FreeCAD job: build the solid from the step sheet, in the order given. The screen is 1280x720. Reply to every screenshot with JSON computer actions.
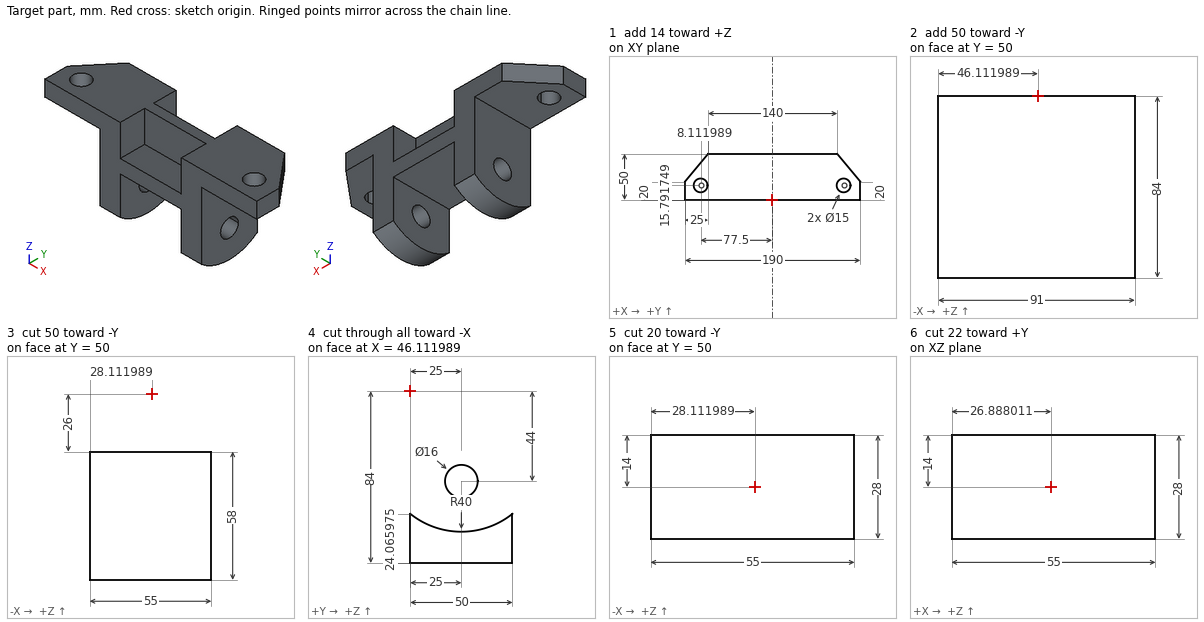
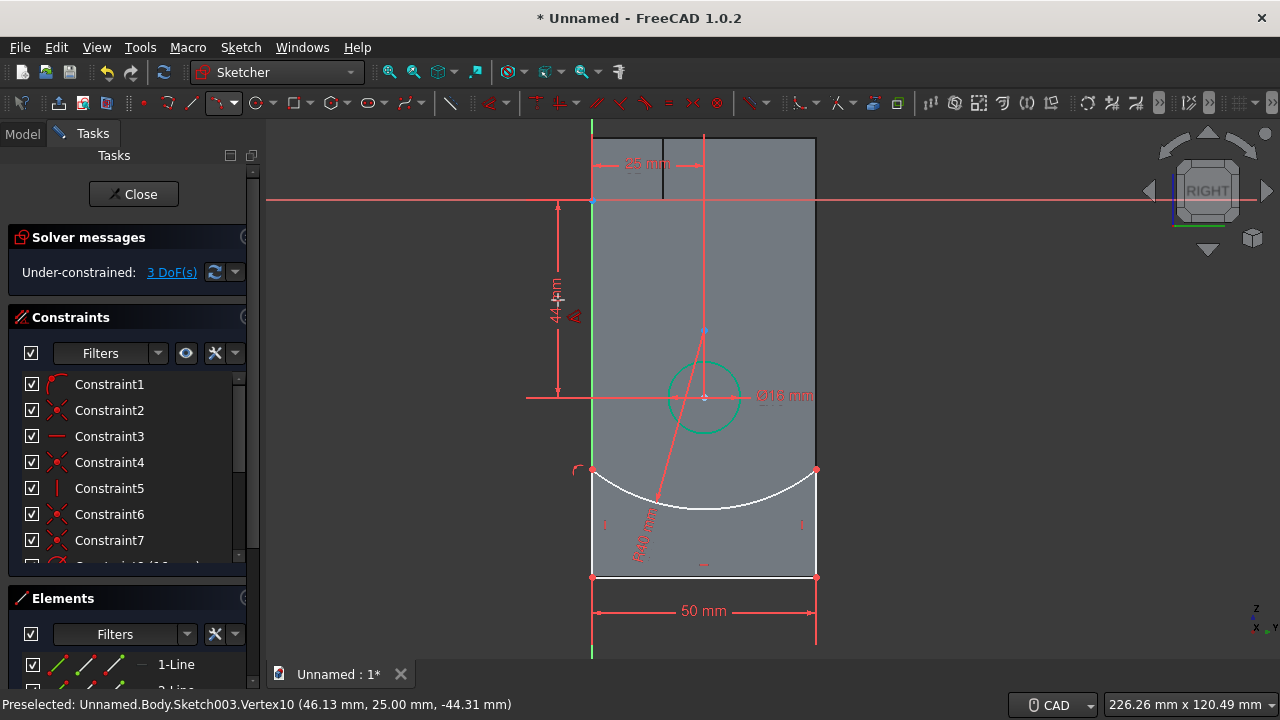
{"action": "left_click", "coordinate": [592, 578]}
{"action": "left_click", "coordinate": [558, 389]}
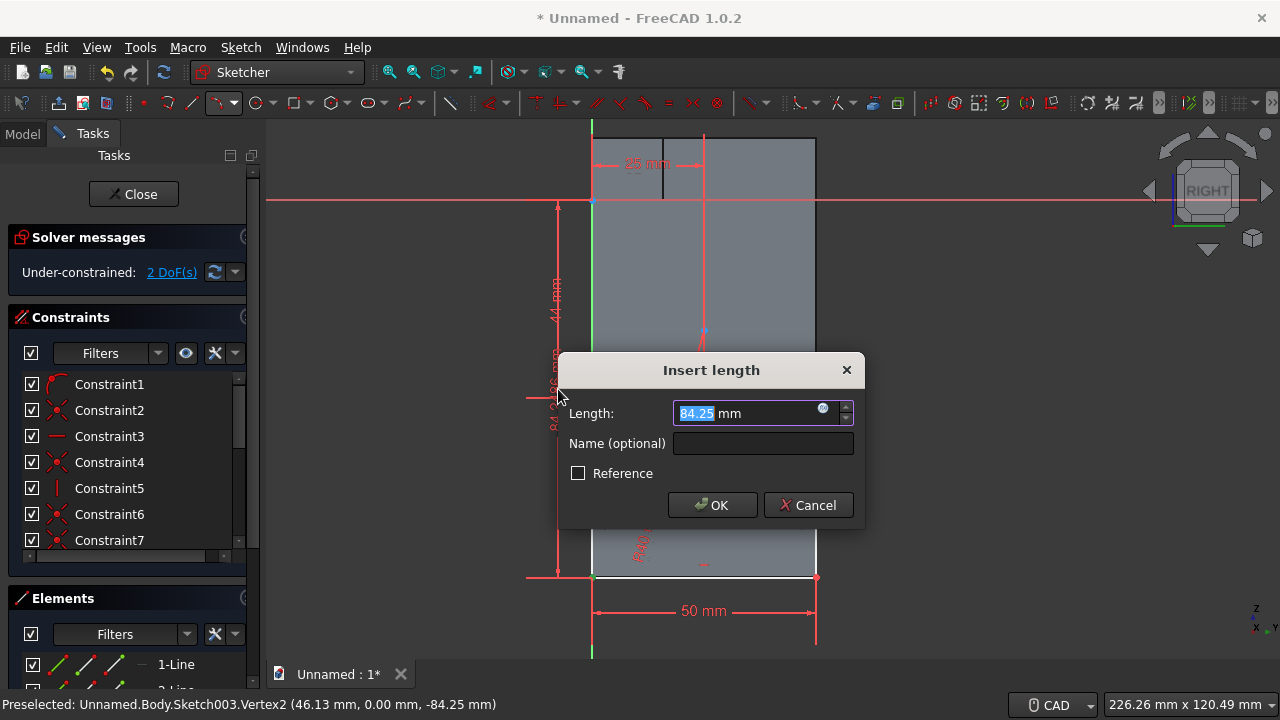
{"action": "type", "text": "84"}
{"action": "key", "text": "Return"}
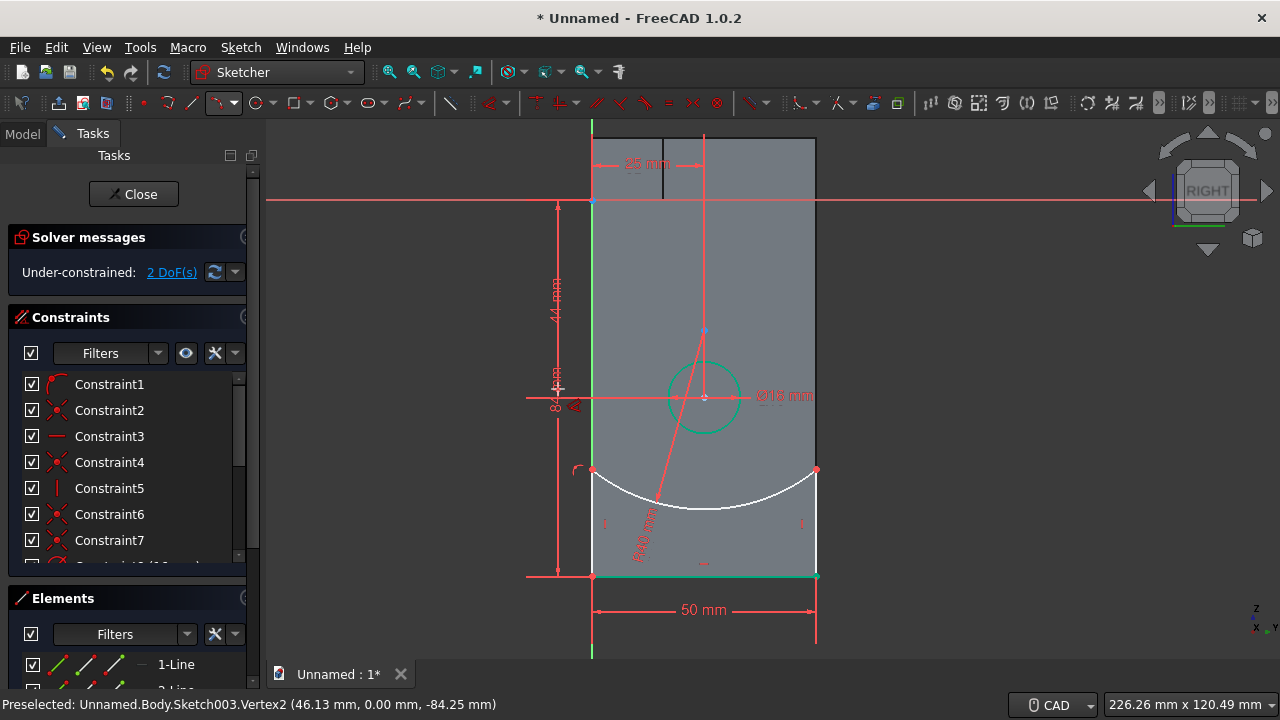
{"action": "left_click", "coordinate": [704, 330]}
{"action": "left_click", "coordinate": [648, 364]}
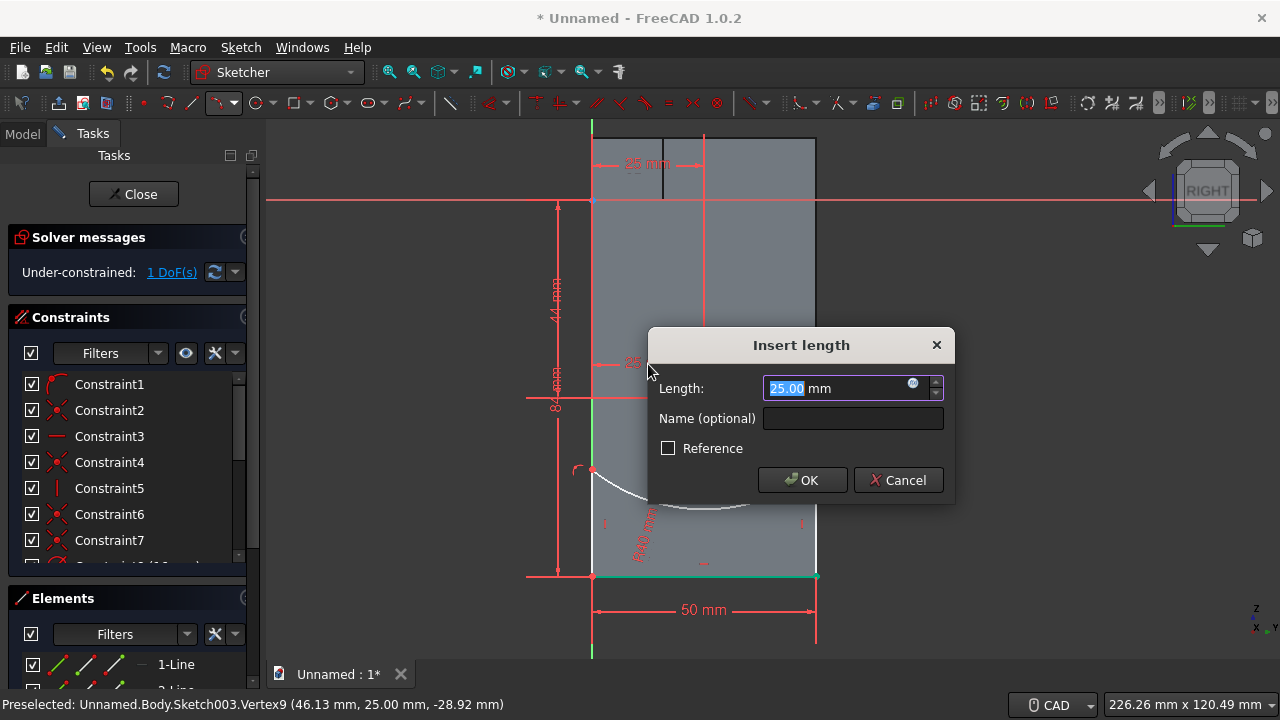
{"action": "type", "text": "25"}
{"action": "key", "text": "Return"}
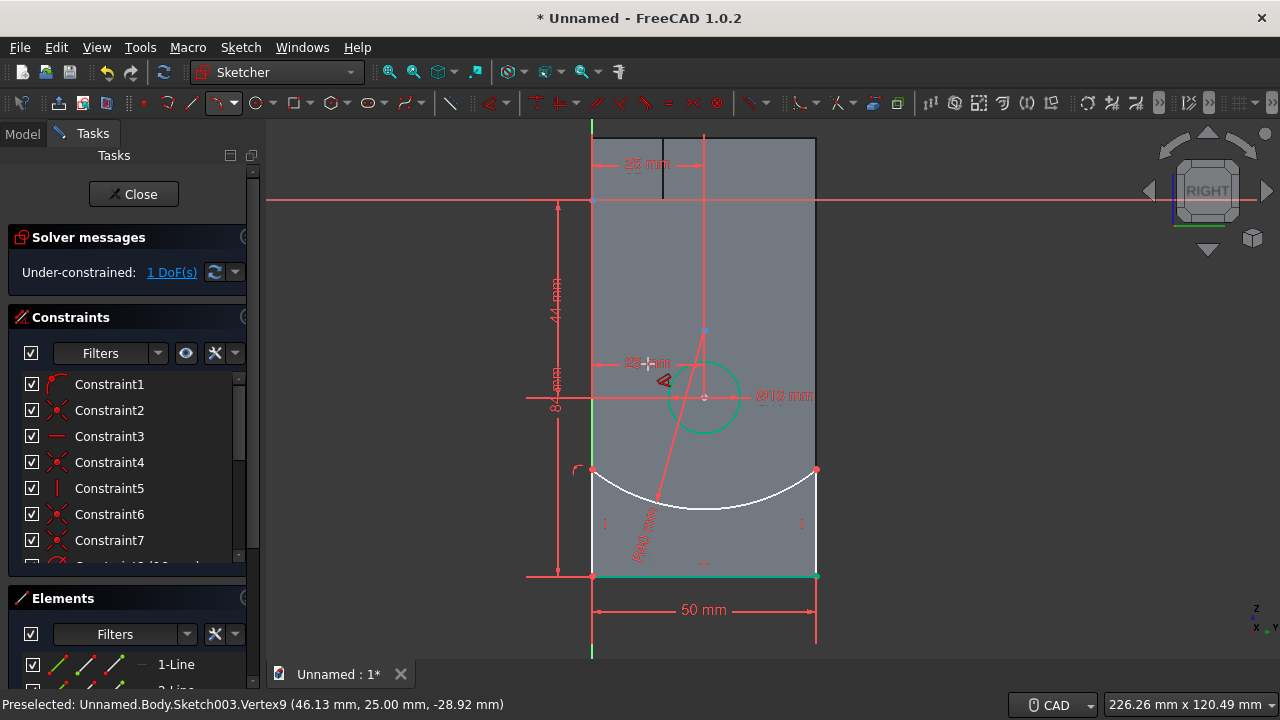
{"action": "left_click", "coordinate": [592, 502]}
{"action": "left_click", "coordinate": [558, 523]}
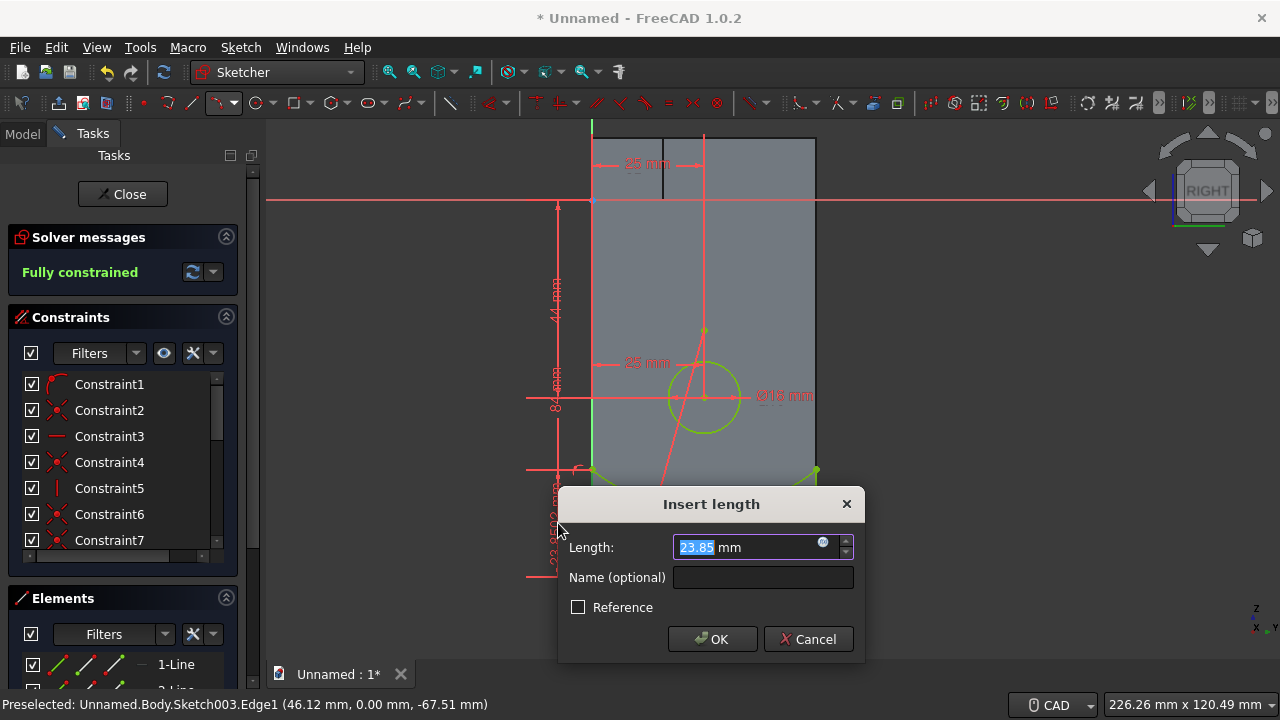
{"action": "type", "text": "24.065975"}
{"action": "key", "text": "Return"}
{"action": "key", "text": "Escape"}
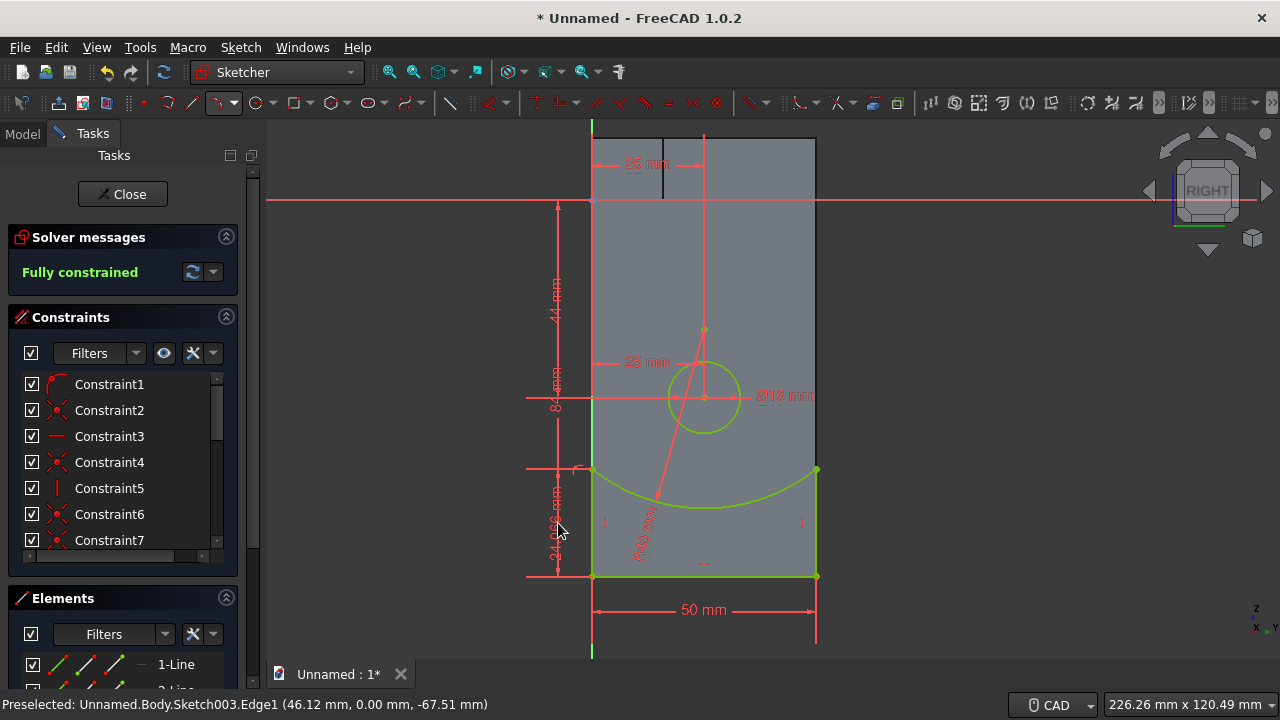
{"action": "left_click", "coordinate": [123, 194]}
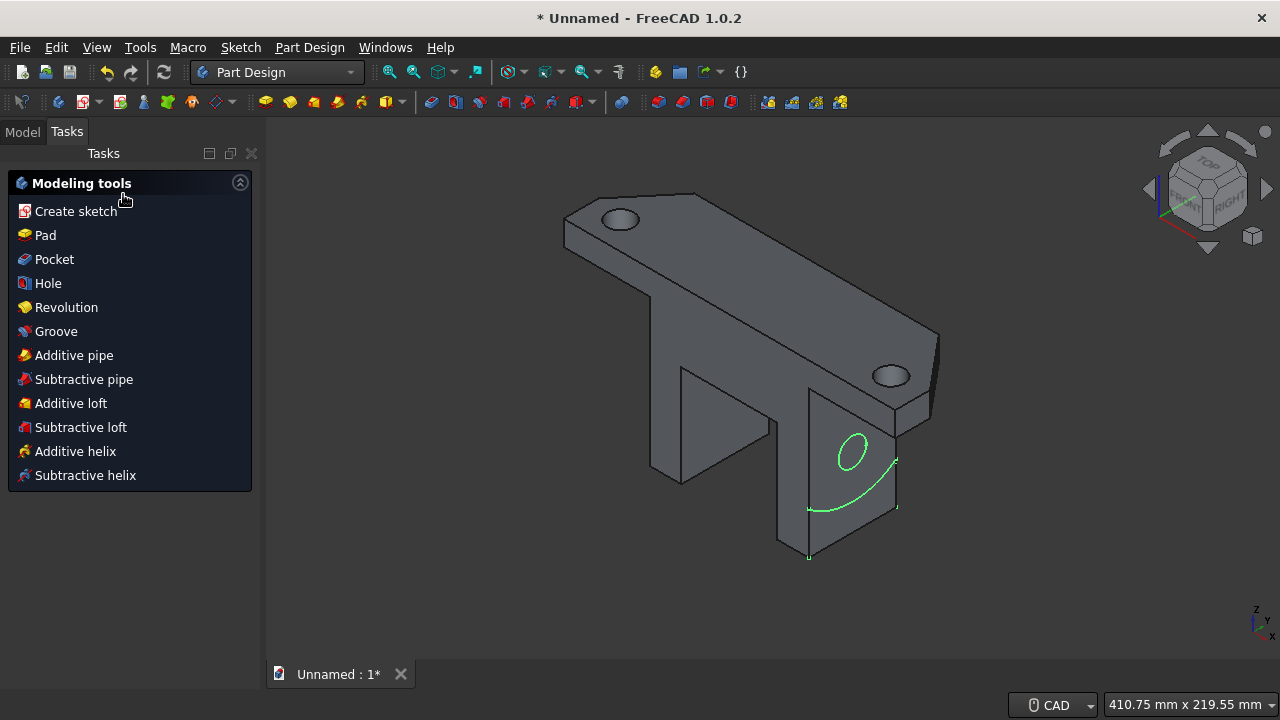
{"action": "left_click", "coordinate": [432, 102]}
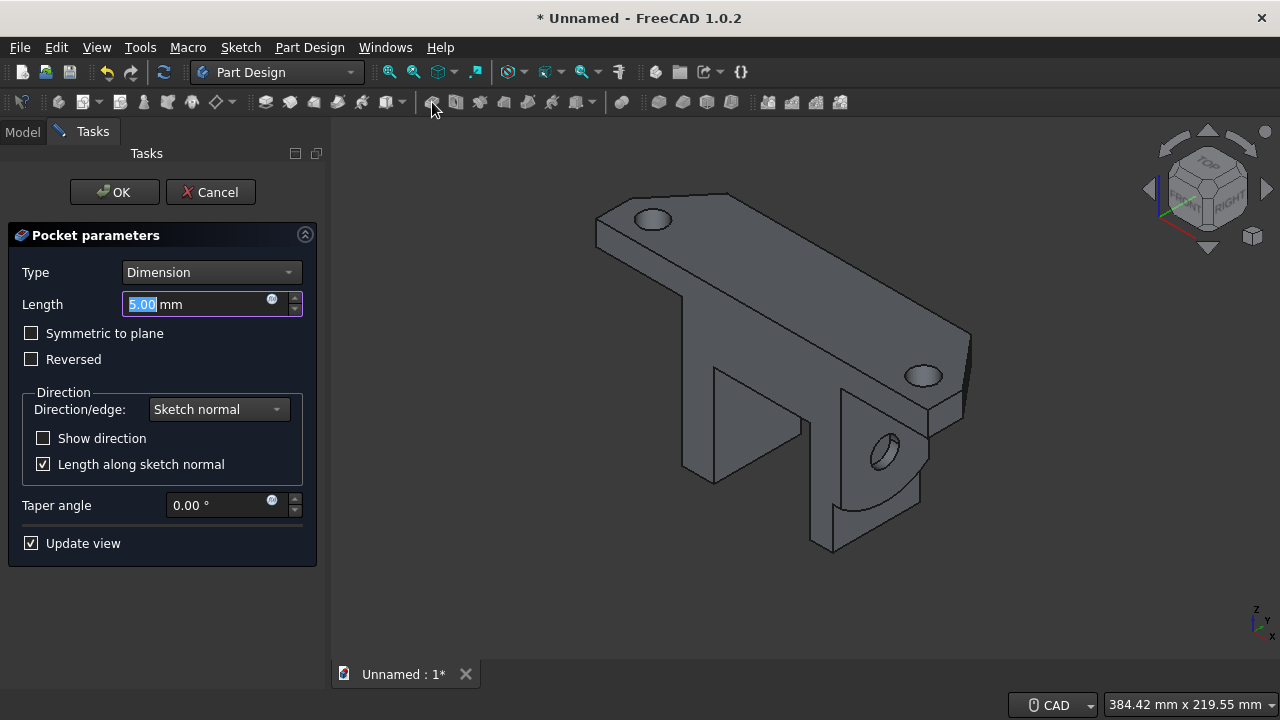
{"action": "left_click", "coordinate": [212, 272]}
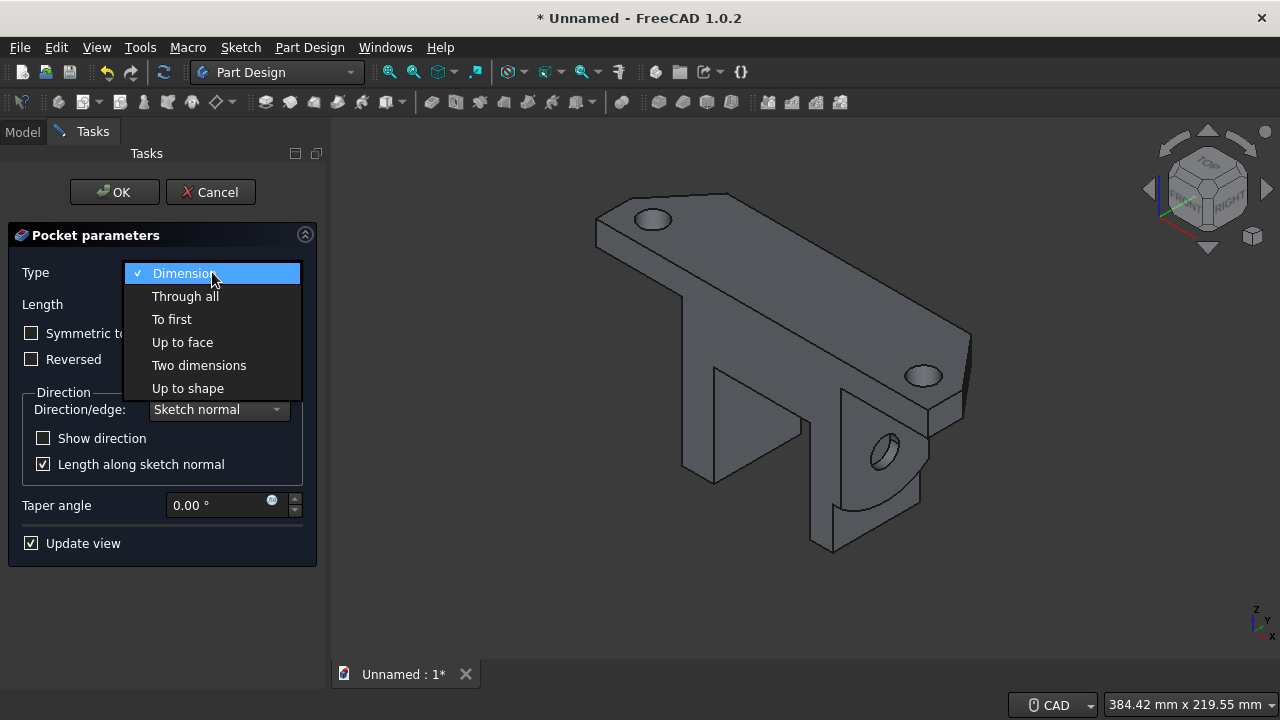
{"action": "left_click", "coordinate": [212, 296]}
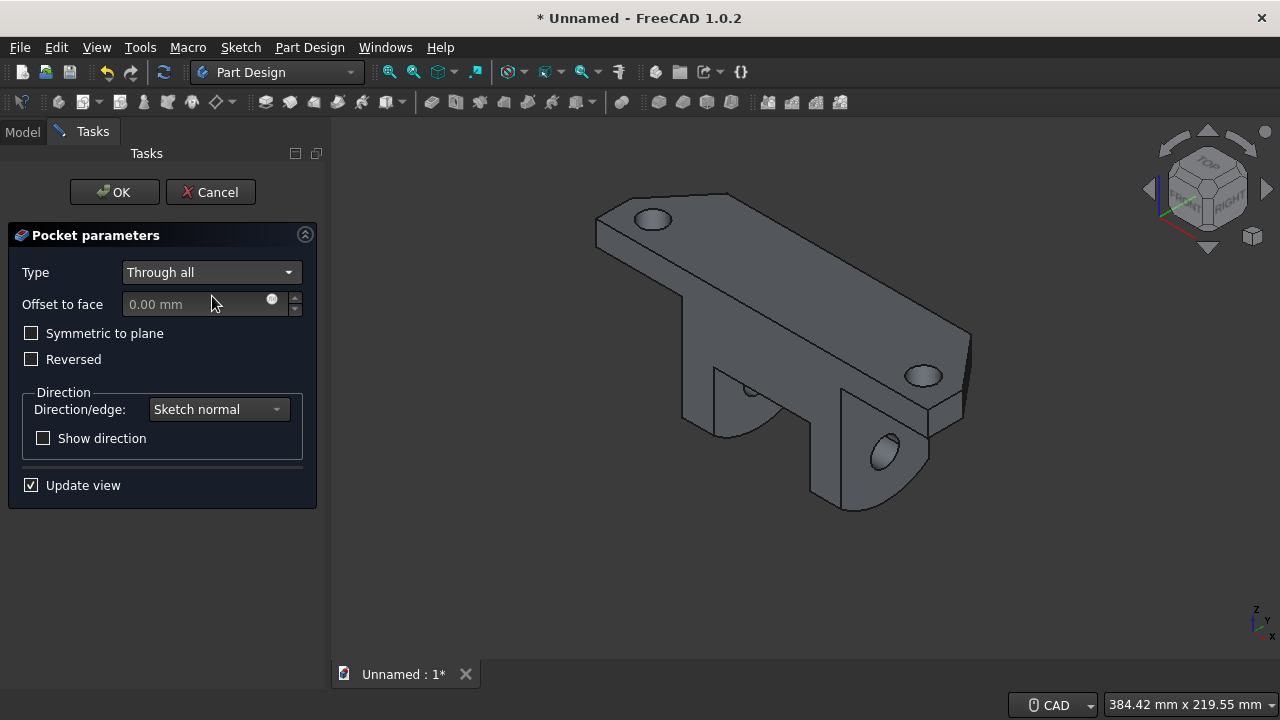
{"action": "left_click", "coordinate": [115, 192]}